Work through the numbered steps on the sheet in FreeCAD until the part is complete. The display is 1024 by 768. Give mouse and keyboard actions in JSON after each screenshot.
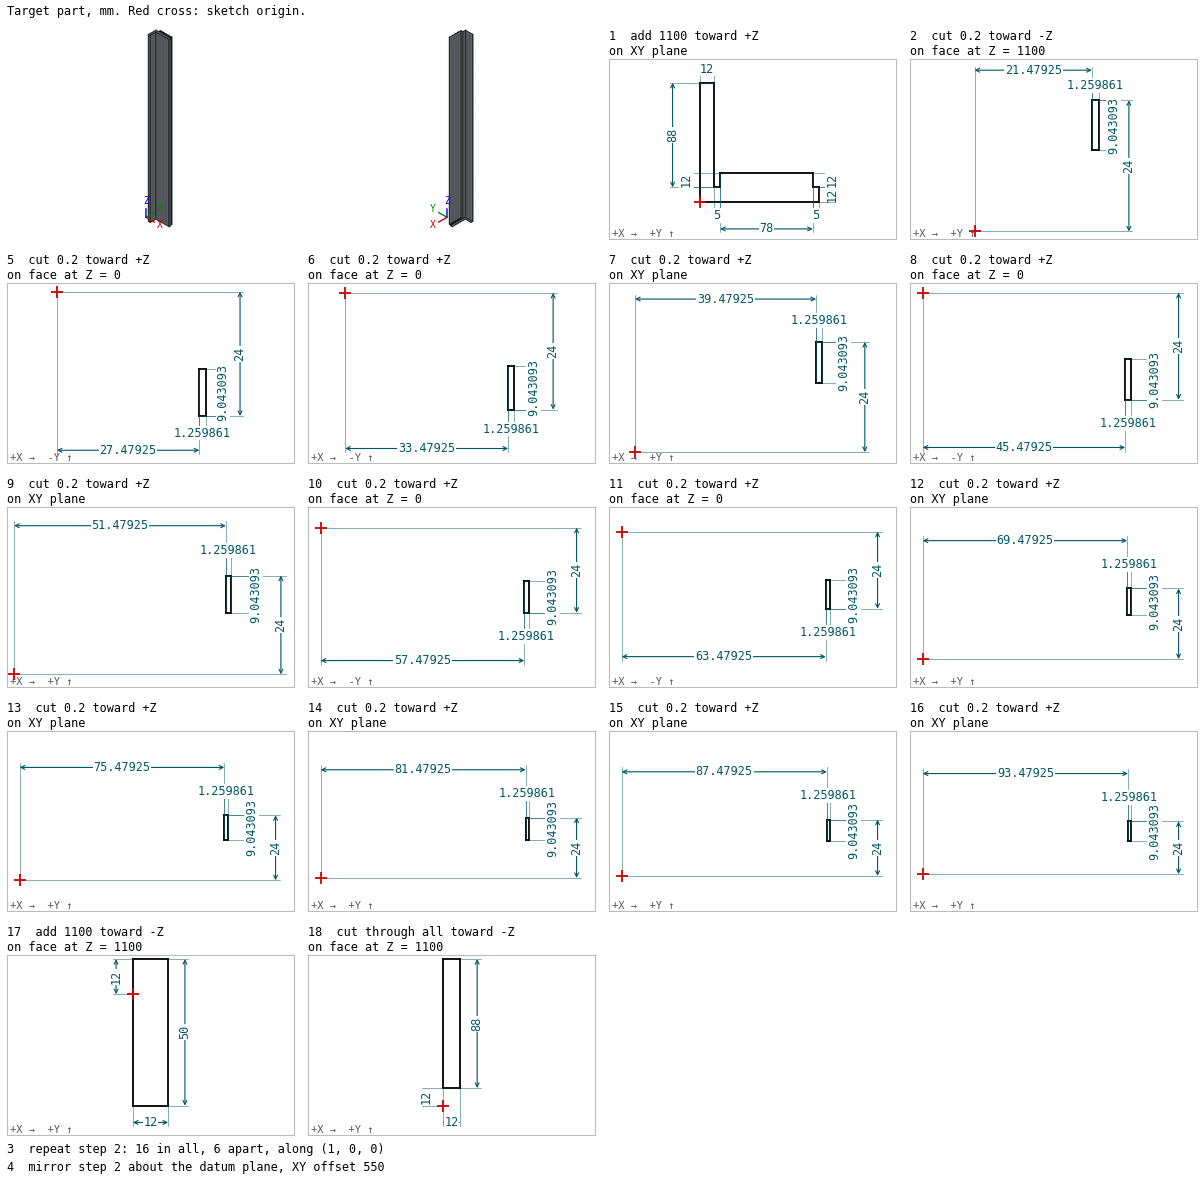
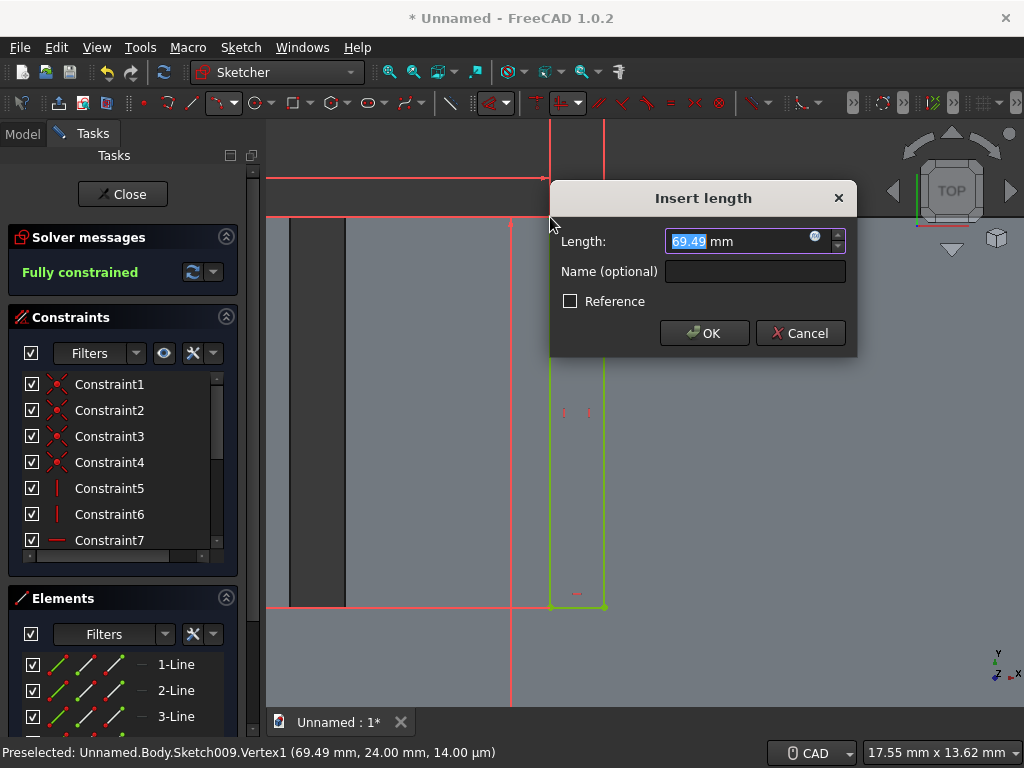
{"action": "type", "text": "69.47925"}
{"action": "key", "text": "Return"}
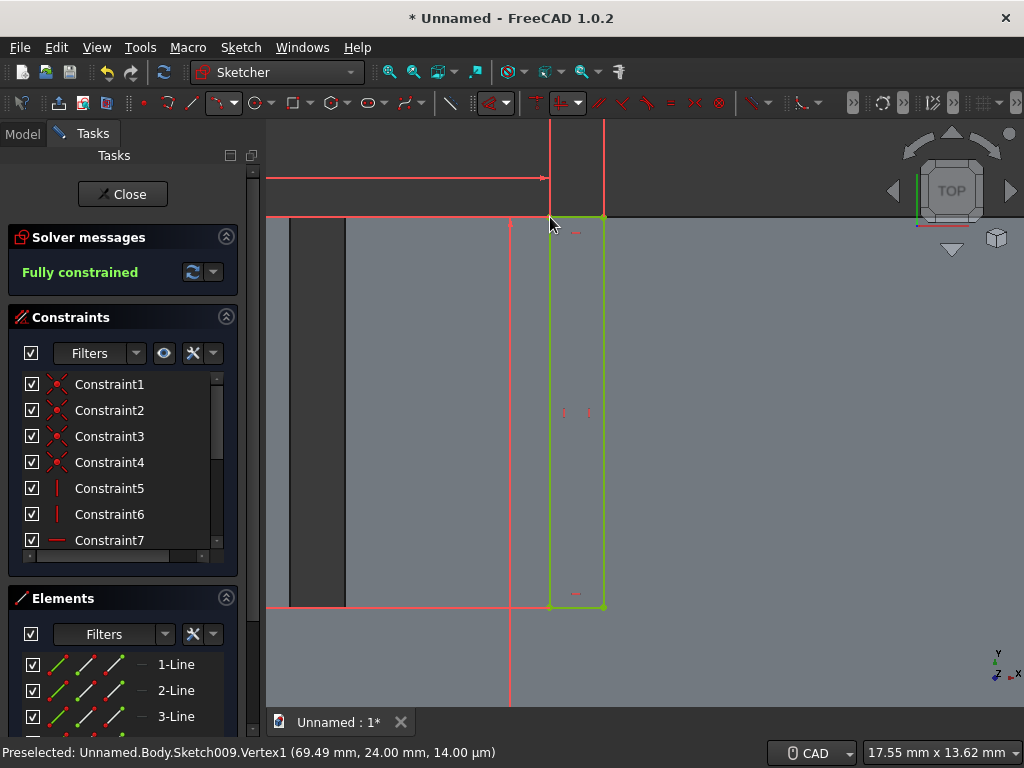
{"action": "left_click", "coordinate": [123, 194]}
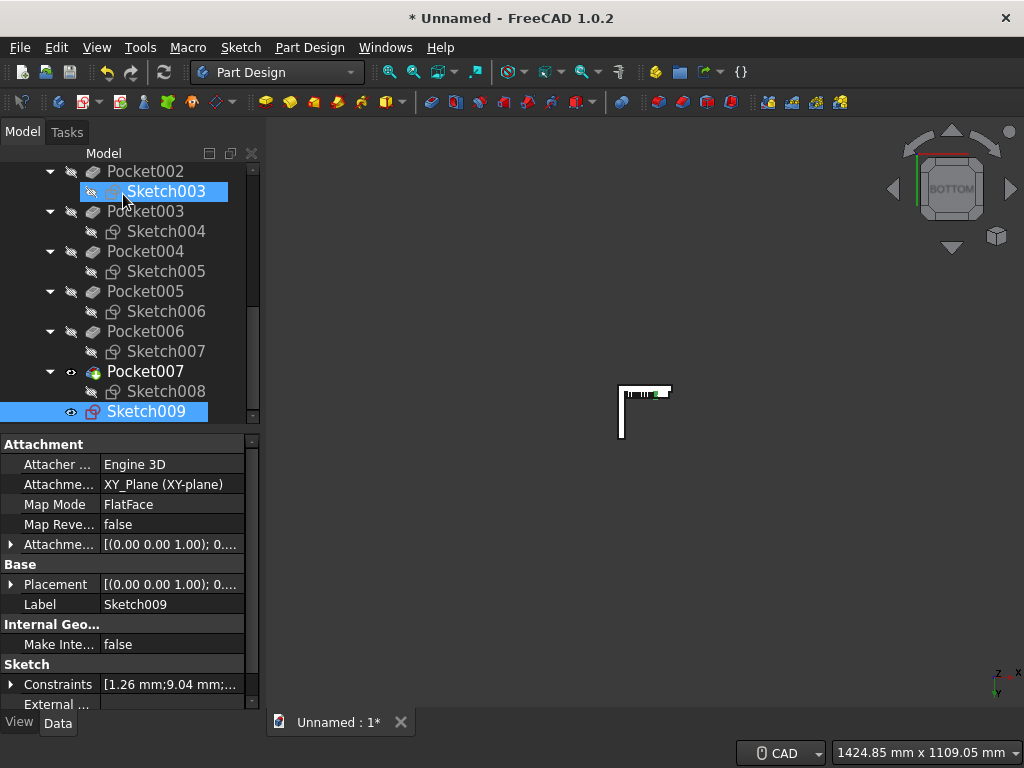
{"action": "left_click", "coordinate": [432, 102]}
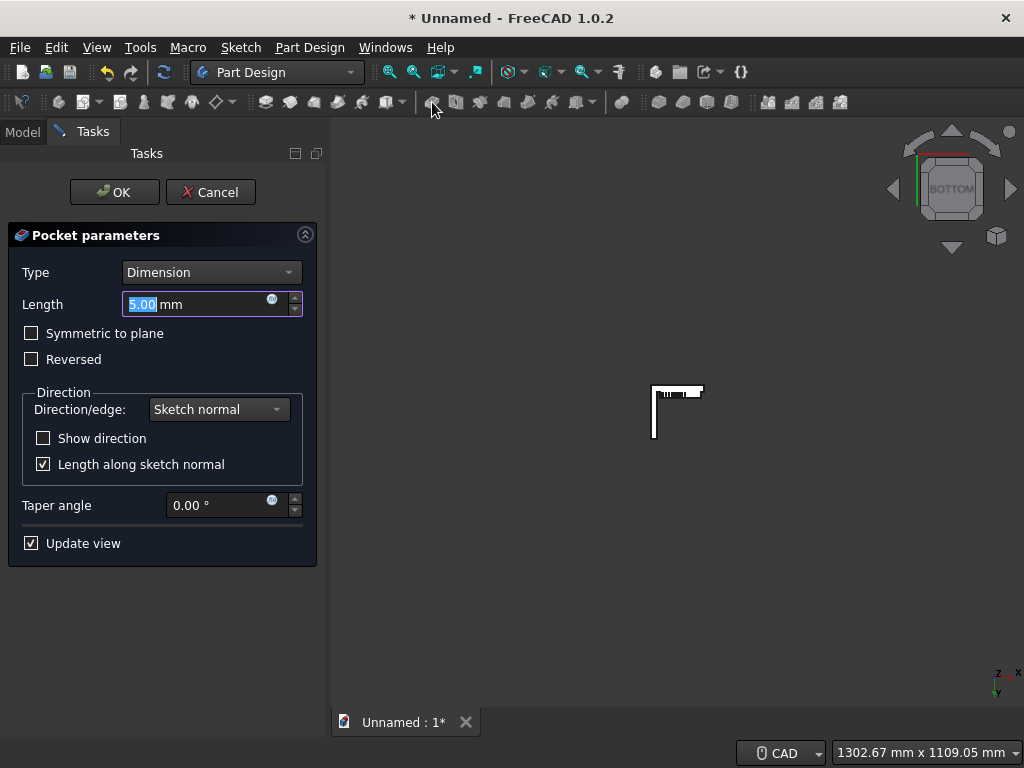
{"action": "type", "text": "0.2"}
{"action": "key", "text": "Tab"}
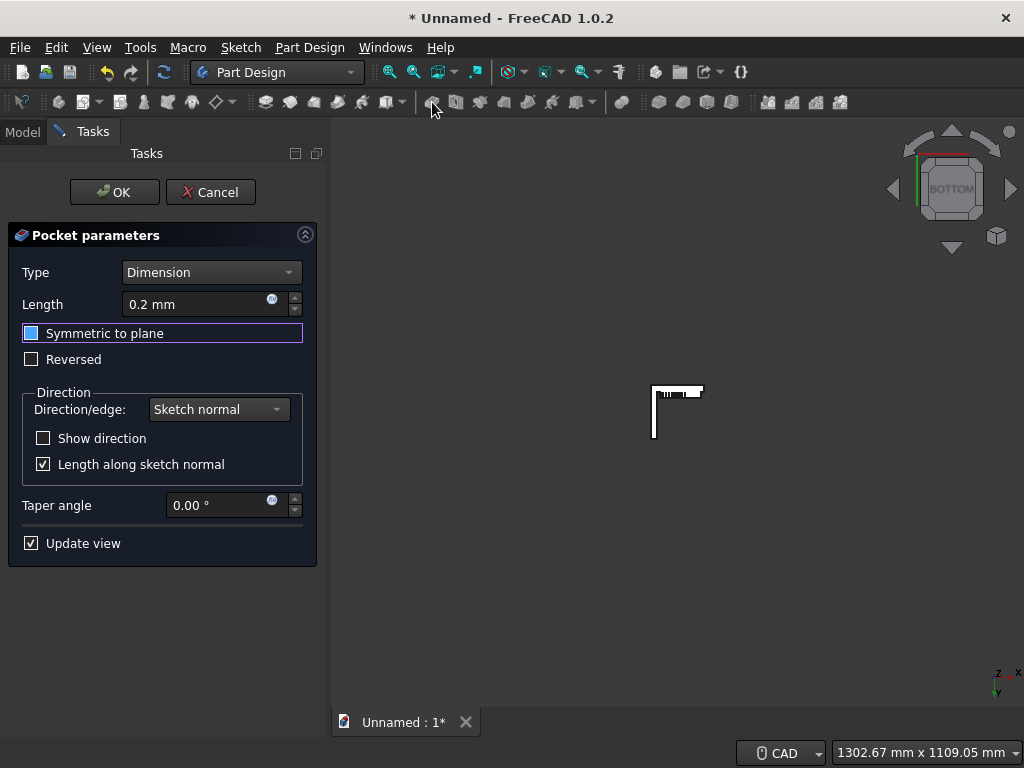
{"action": "left_click", "coordinate": [30, 359]}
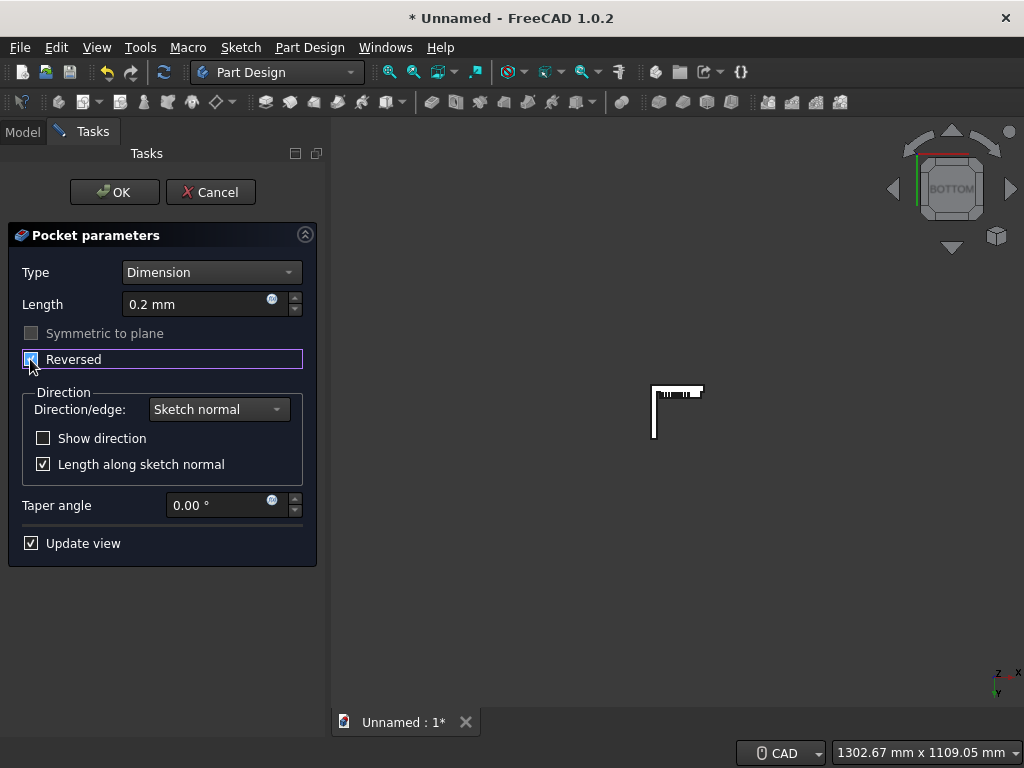
{"action": "left_click", "coordinate": [115, 192]}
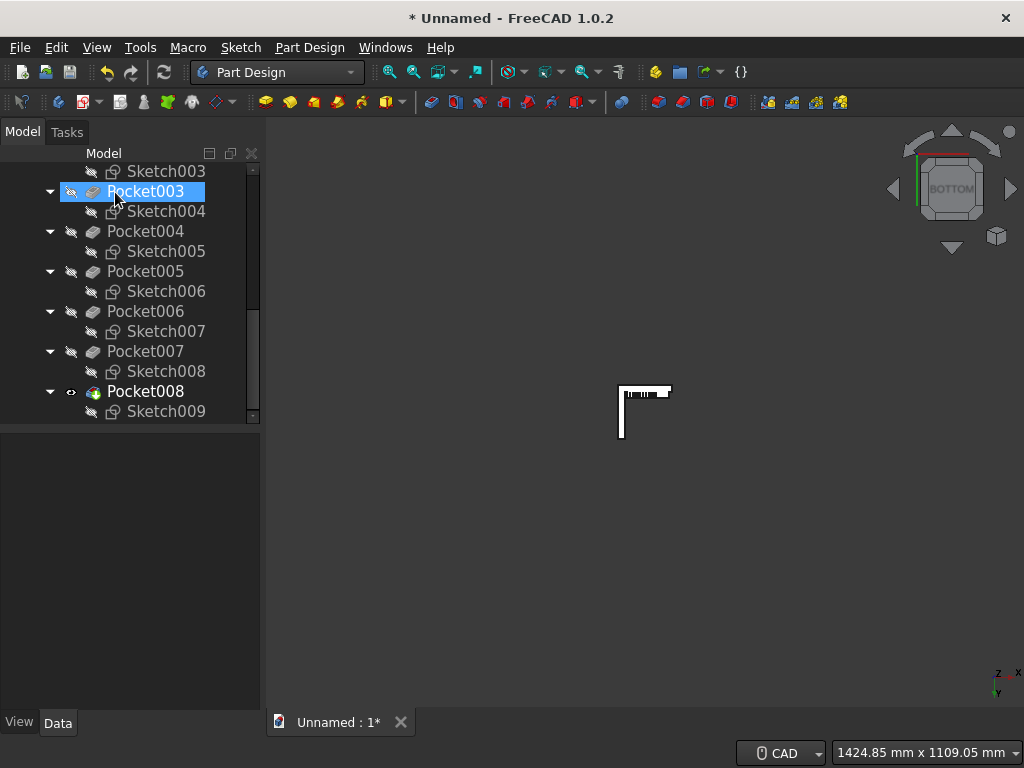
{"action": "left_click", "coordinate": [390, 72]}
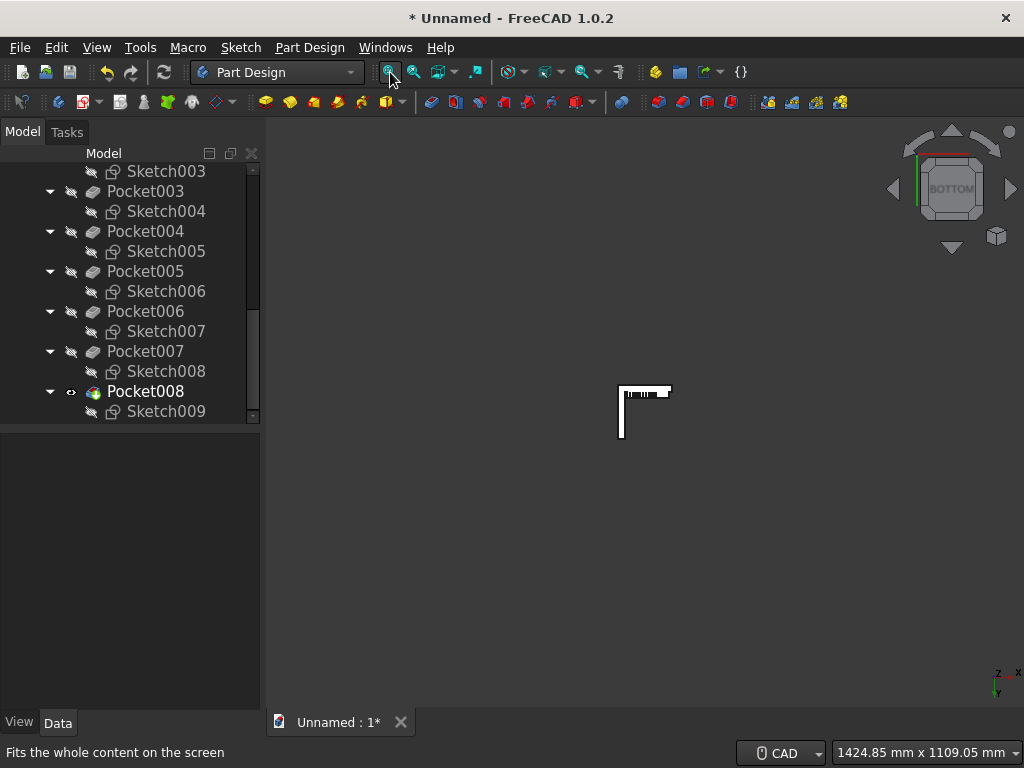
{"action": "left_click", "coordinate": [84, 102]}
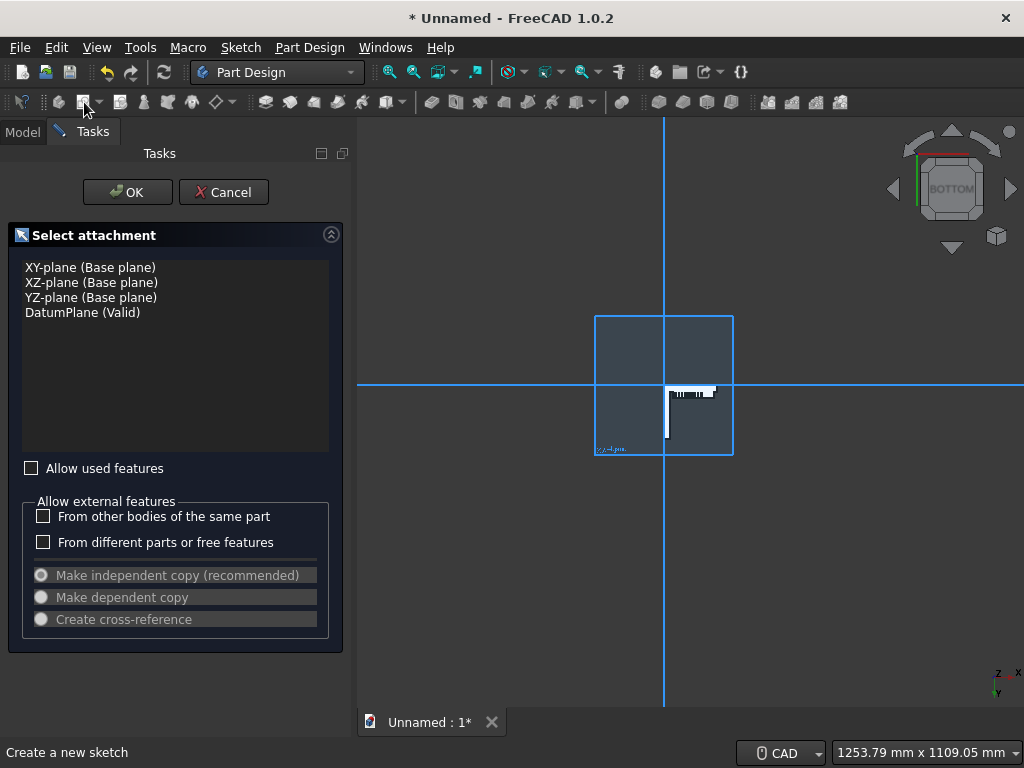
{"action": "left_click", "coordinate": [82, 268]}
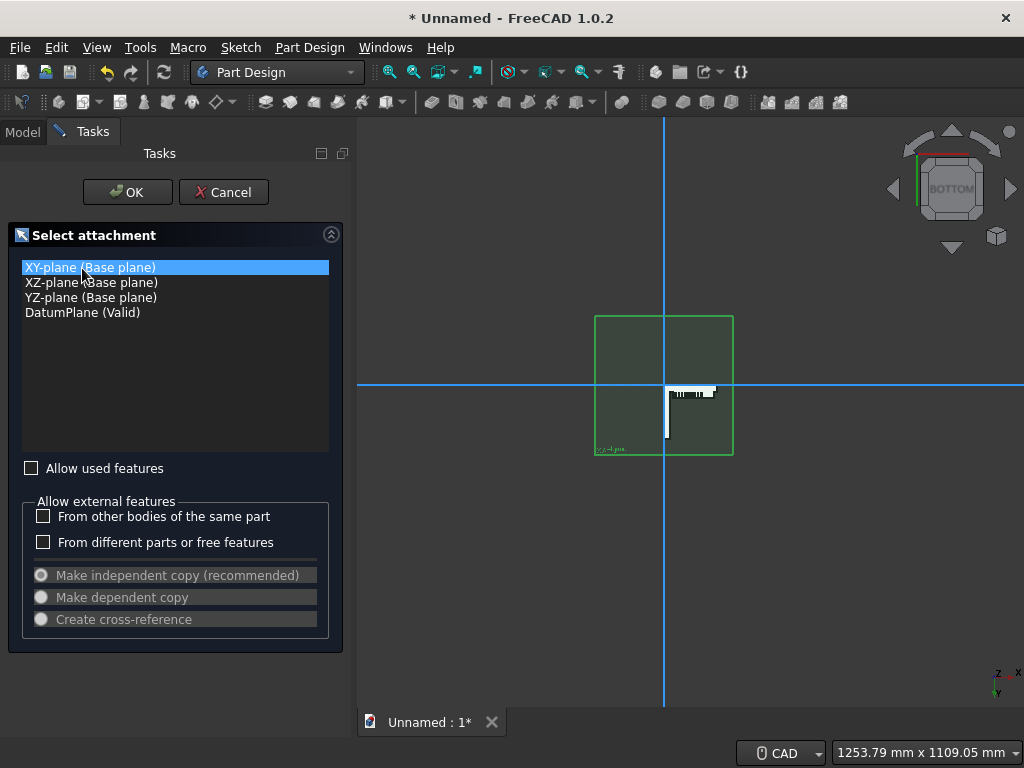
{"action": "left_click", "coordinate": [128, 192]}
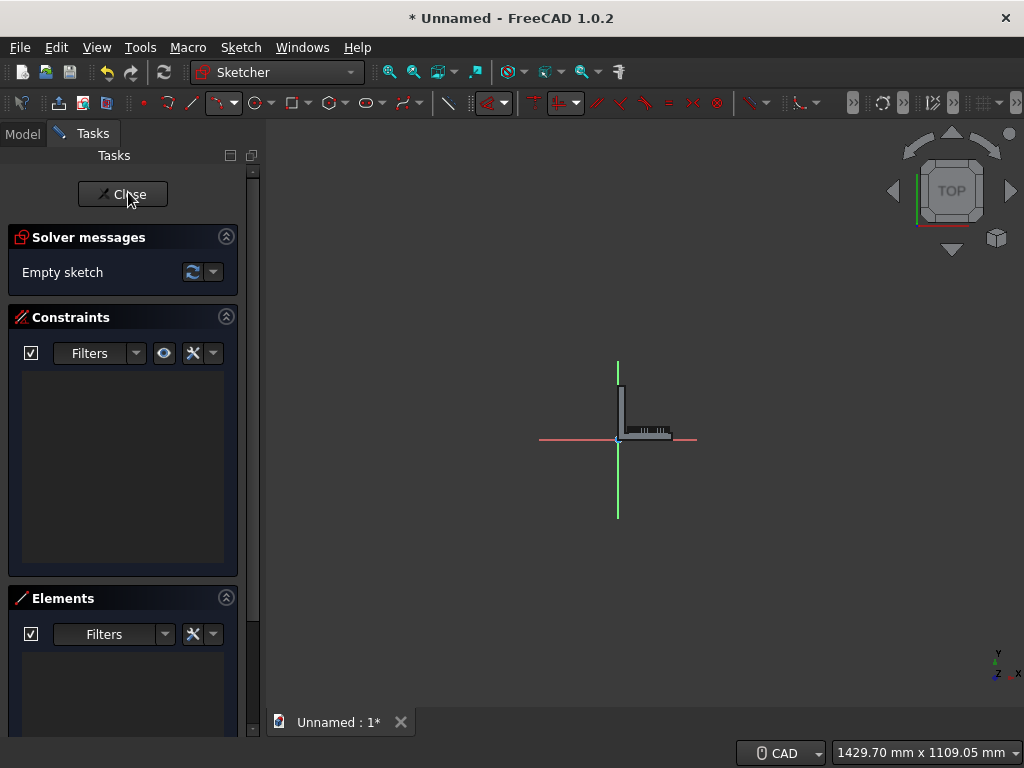
{"action": "key", "text": "q s"}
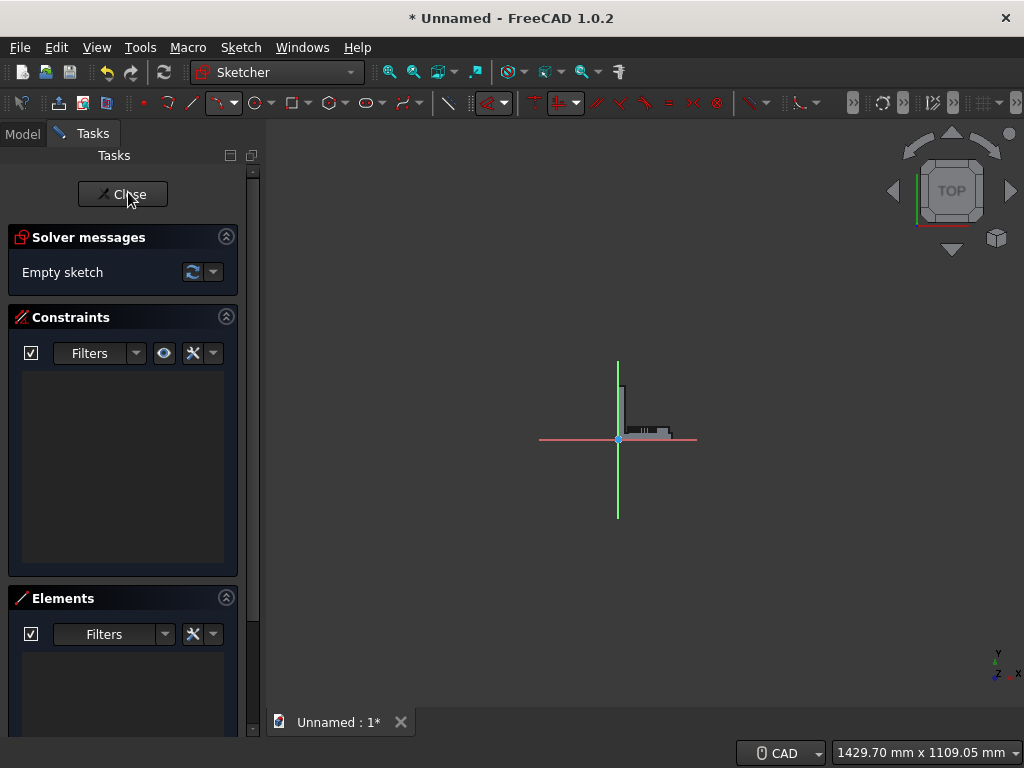
{"action": "scroll", "coordinate": [663, 430], "scroll_direction": "up", "scroll_amount": 15}